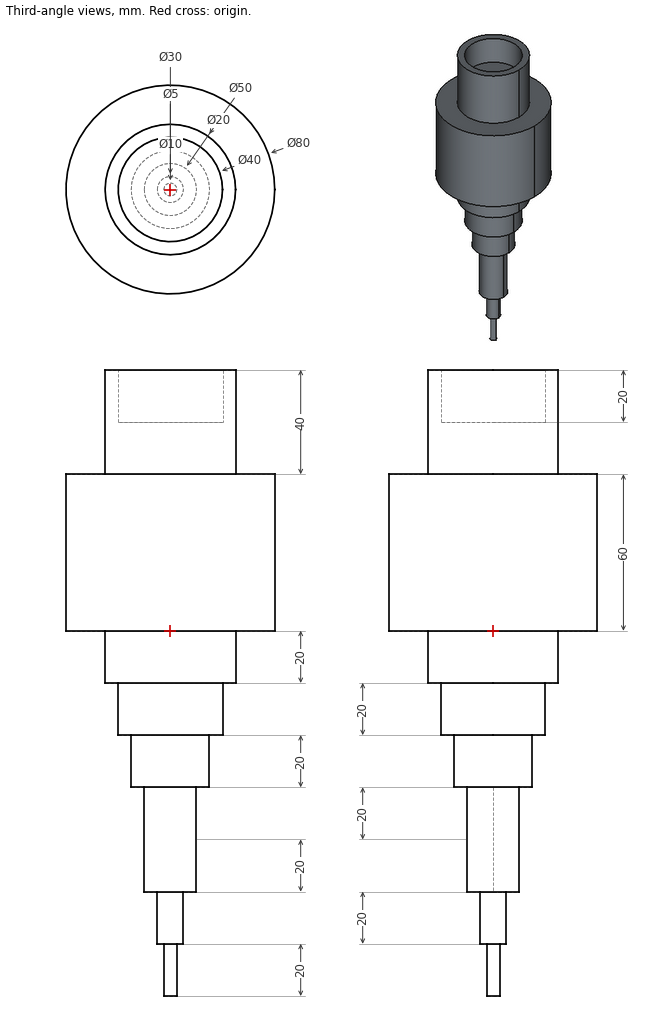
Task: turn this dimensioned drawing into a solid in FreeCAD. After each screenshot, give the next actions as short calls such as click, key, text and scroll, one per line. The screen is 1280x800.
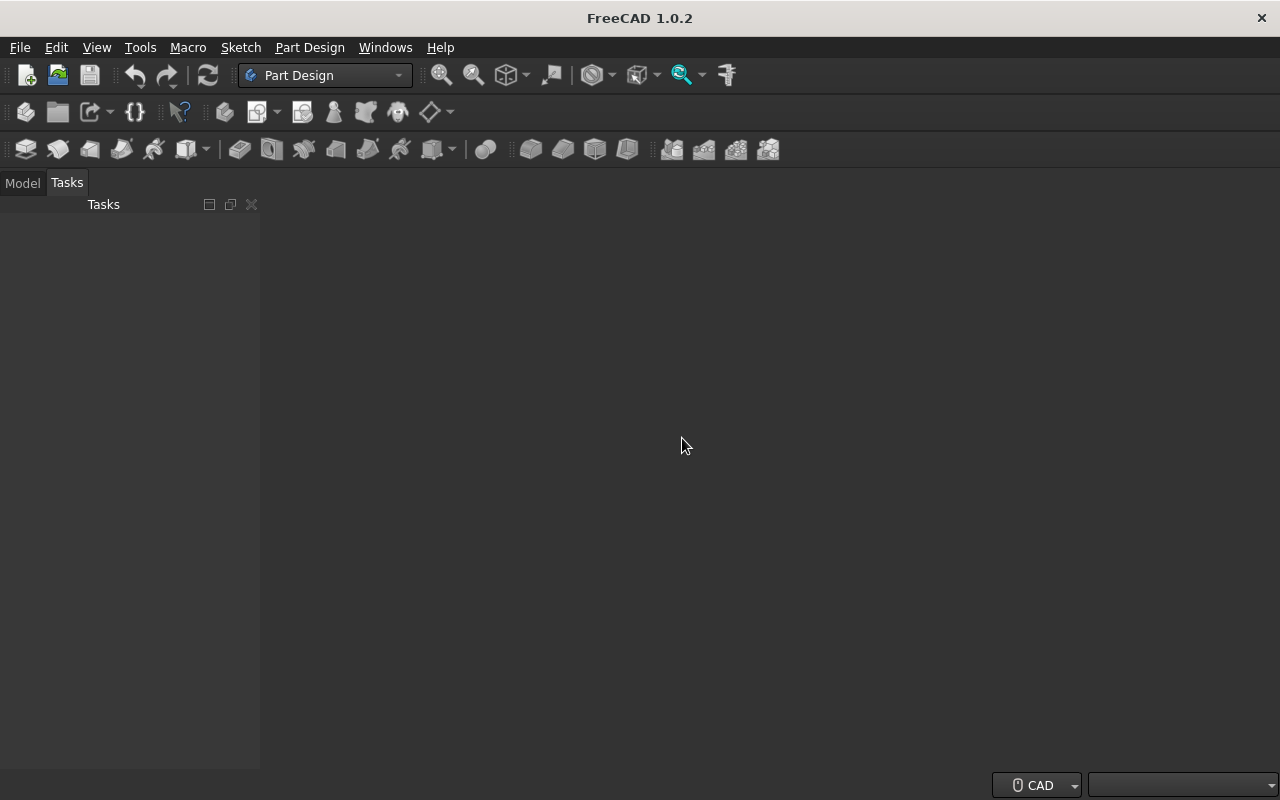
click(26, 76)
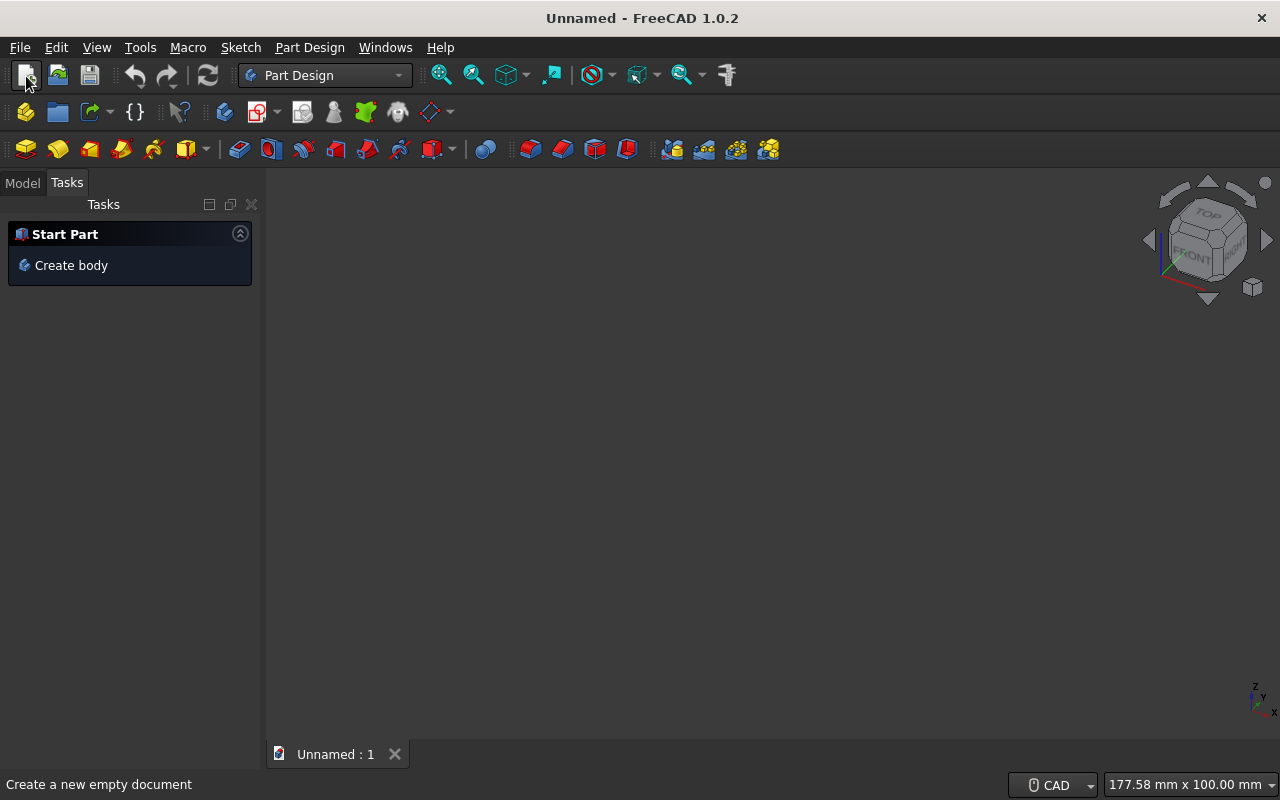
click(258, 112)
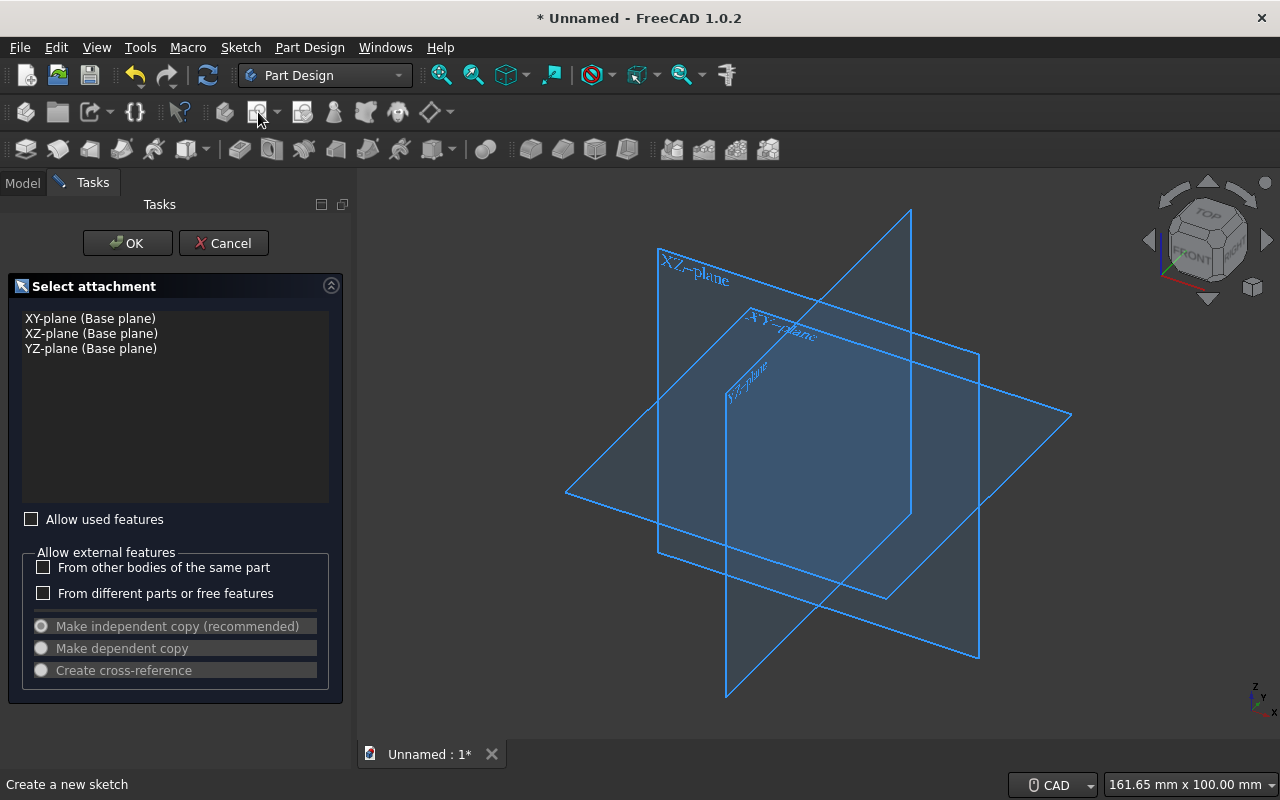
click(82, 318)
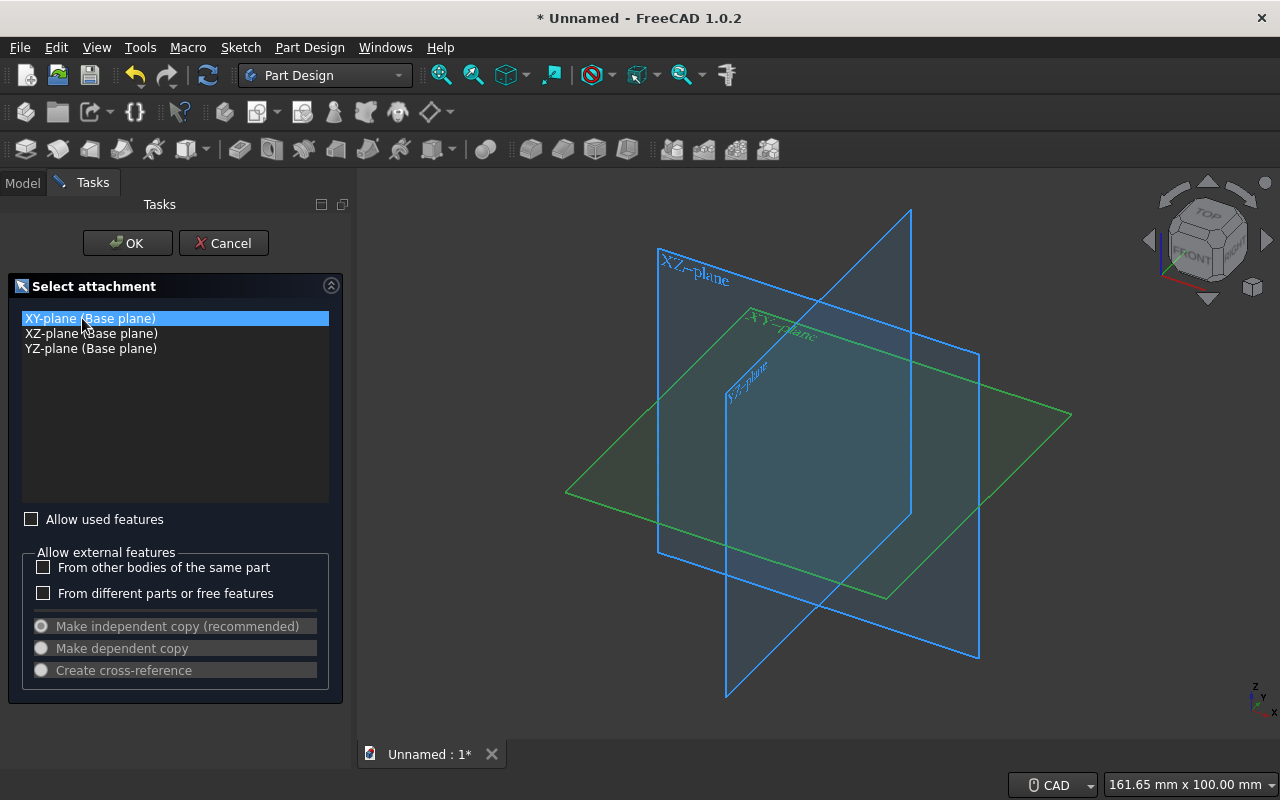
click(128, 243)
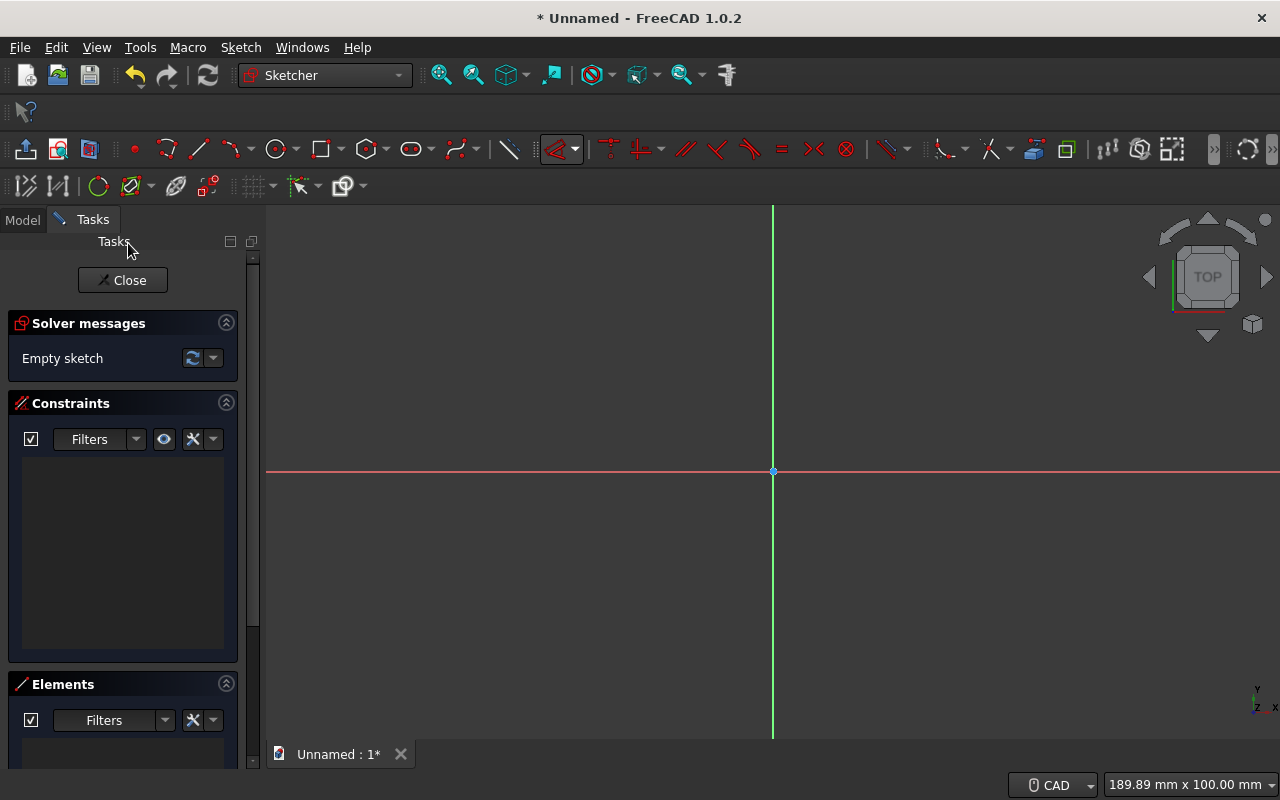
click(276, 150)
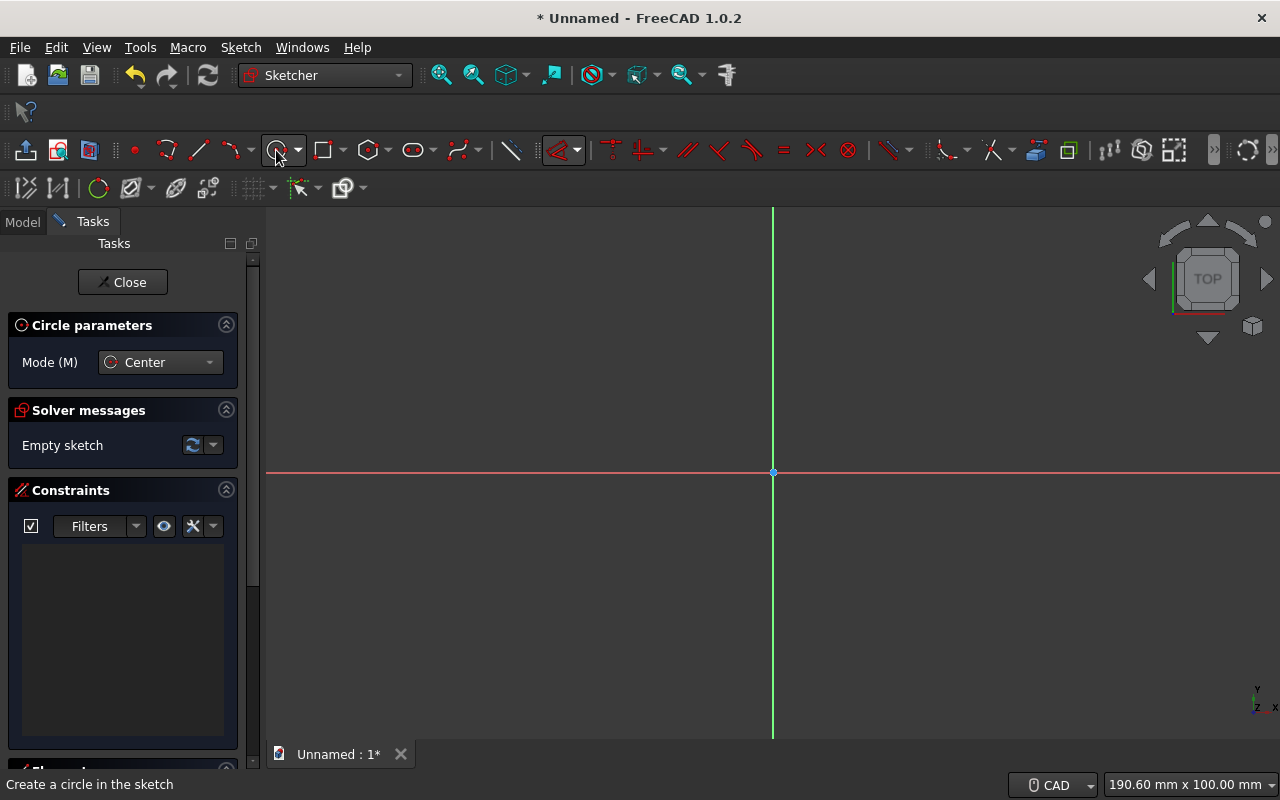
click(773, 473)
click(923, 323)
key(Escape)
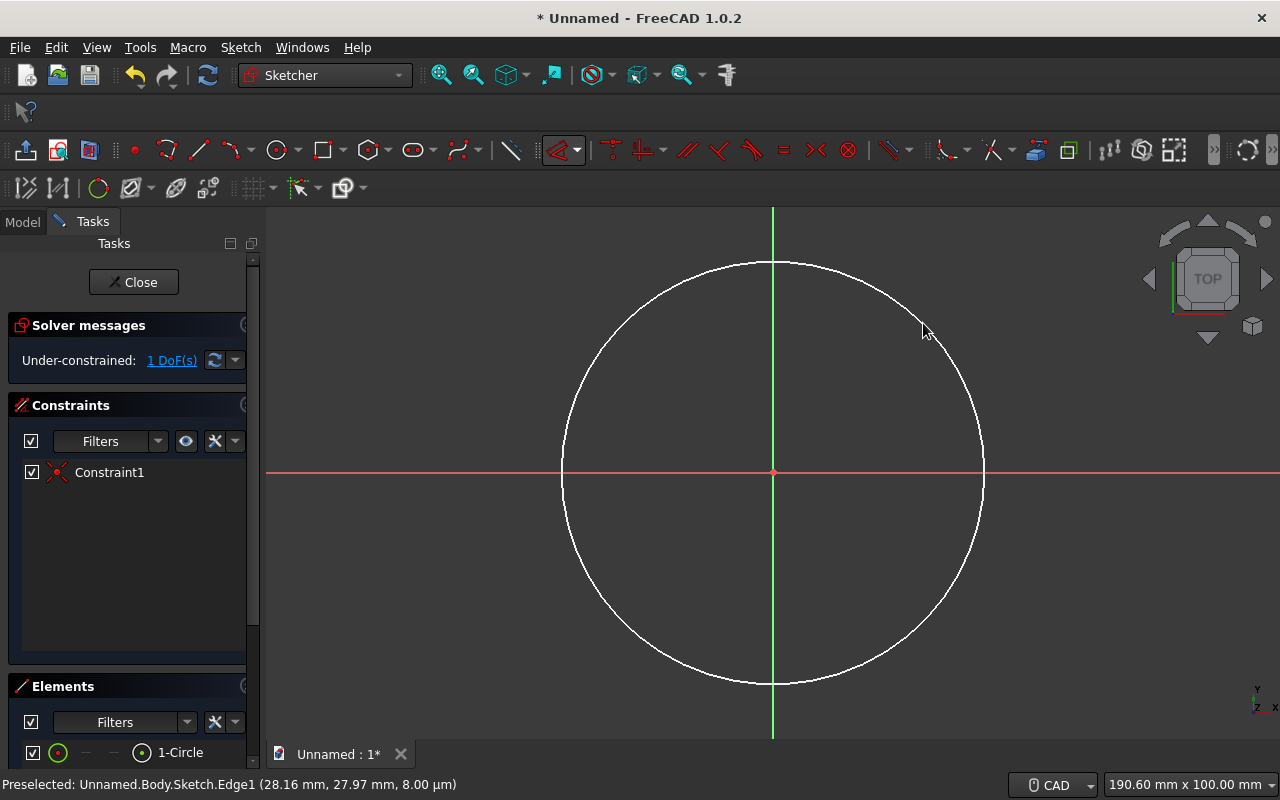
click(558, 150)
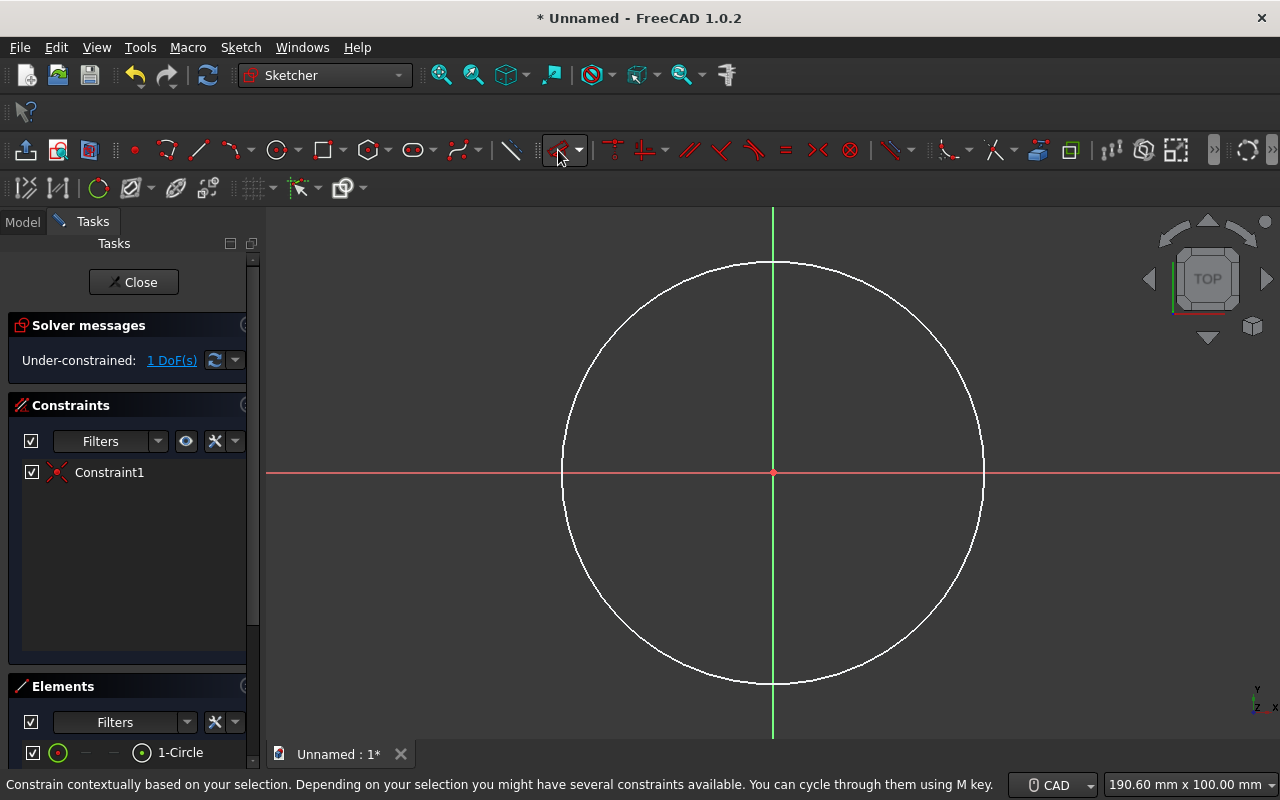
click(922, 323)
click(945, 300)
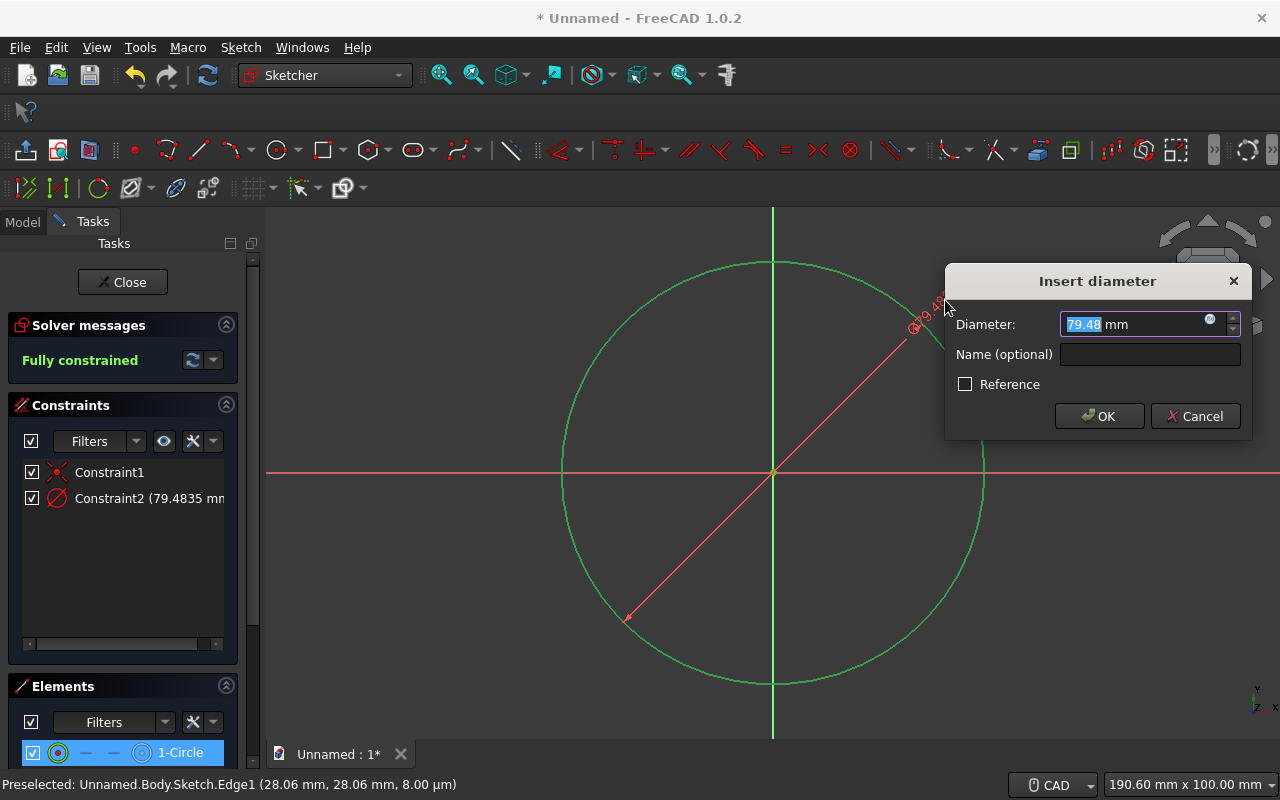
text(80)
key(Return)
key(Escape)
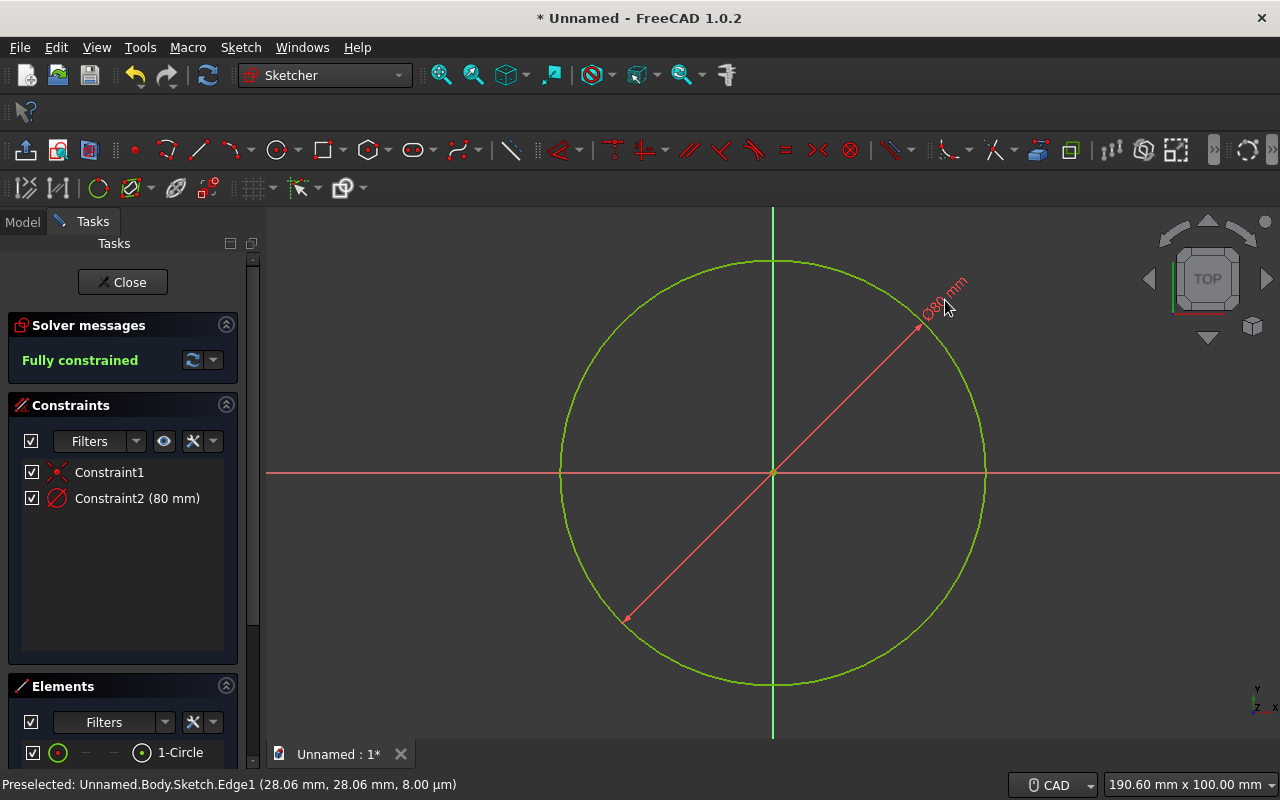
click(123, 282)